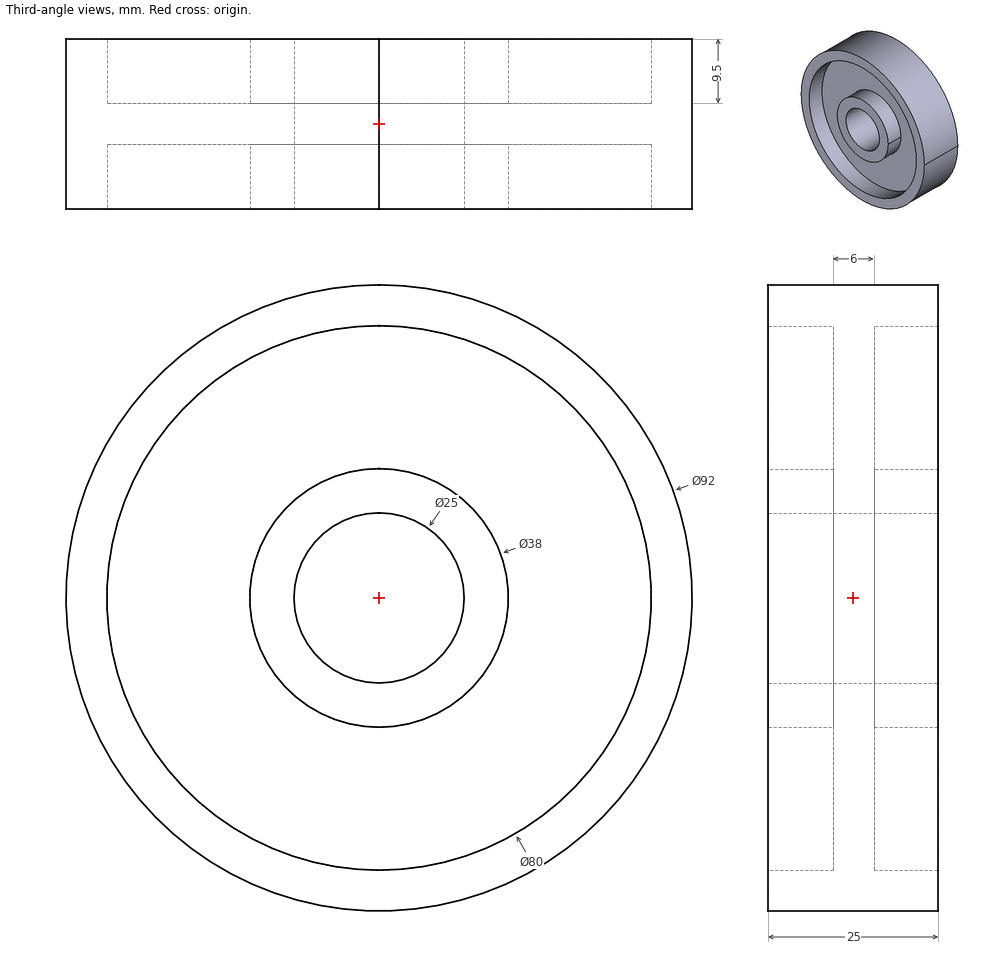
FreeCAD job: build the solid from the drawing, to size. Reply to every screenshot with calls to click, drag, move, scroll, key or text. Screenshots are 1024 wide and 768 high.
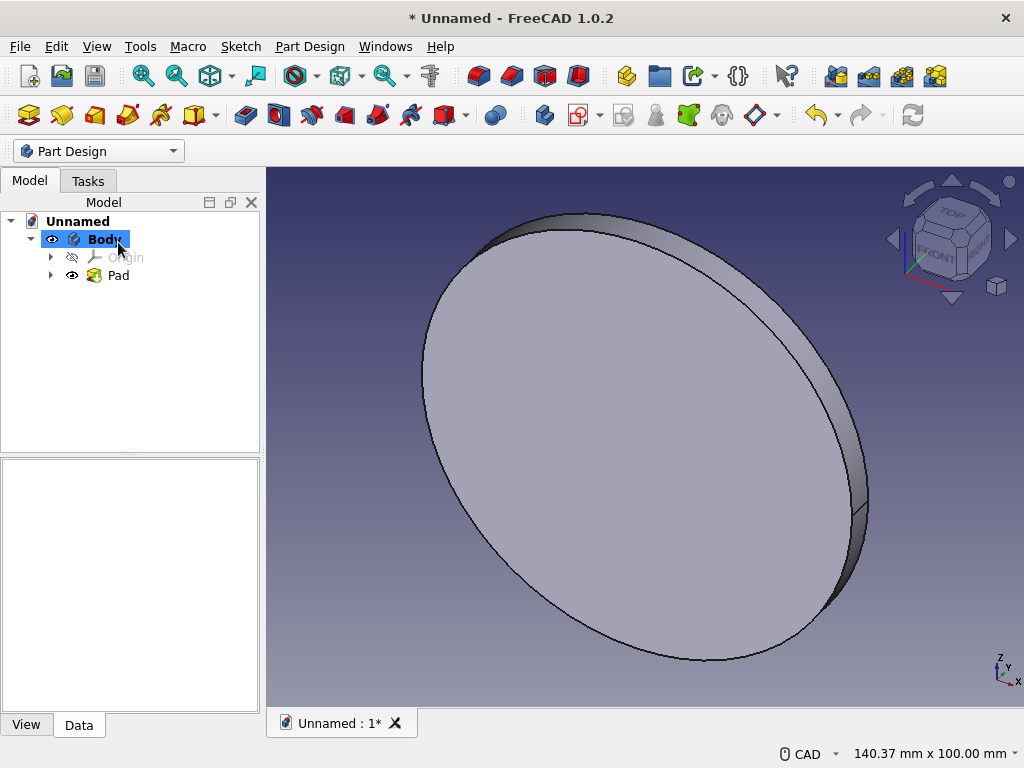
key(v)
key(f)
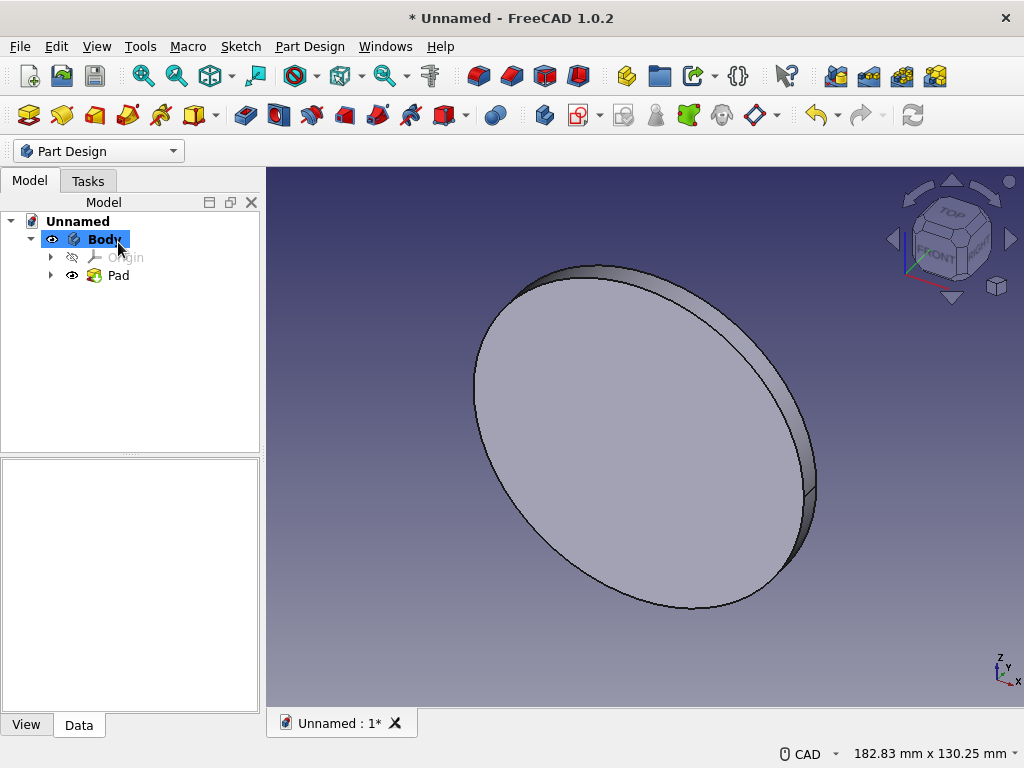
click(51, 257)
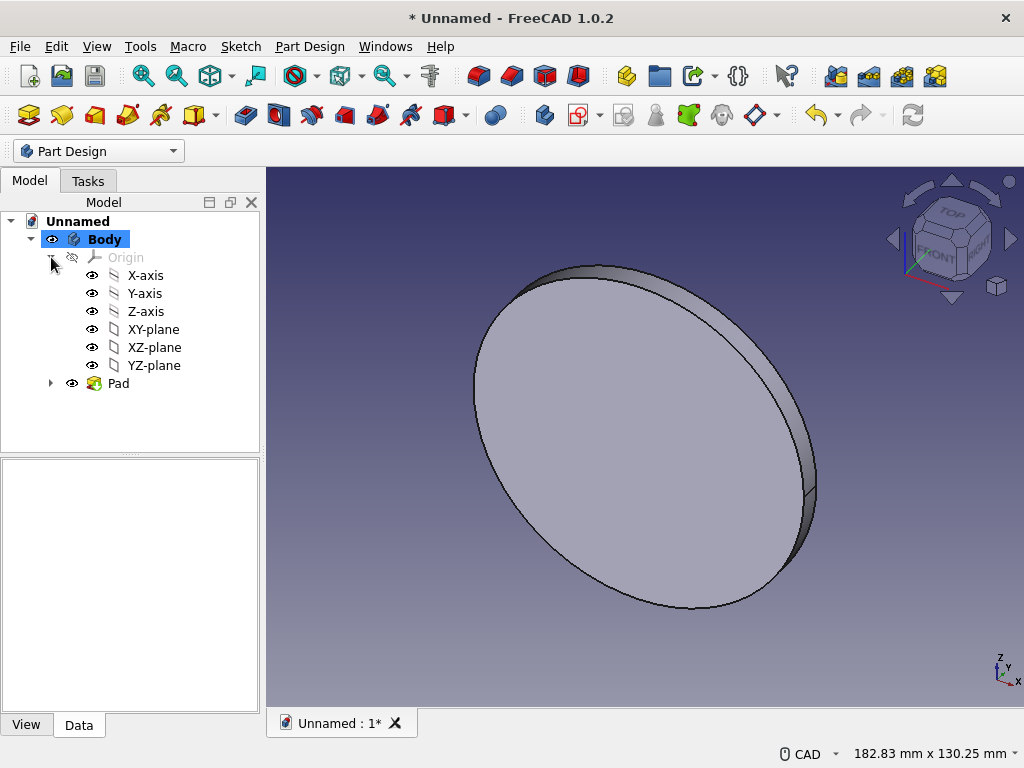
click(137, 347)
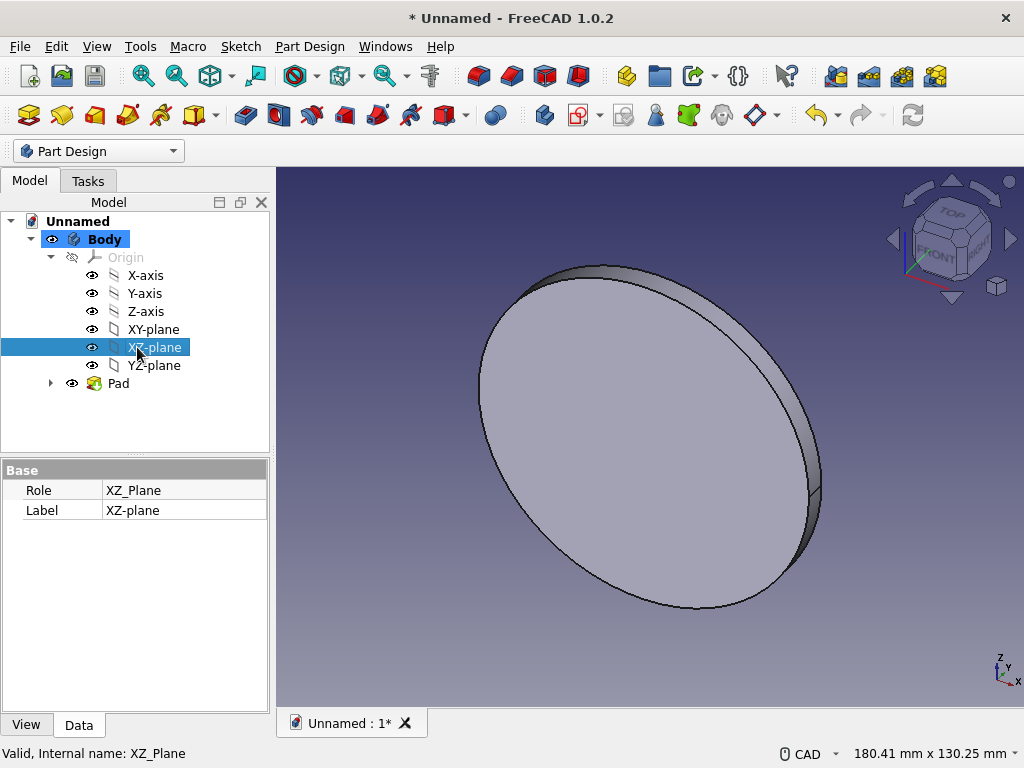
click(754, 116)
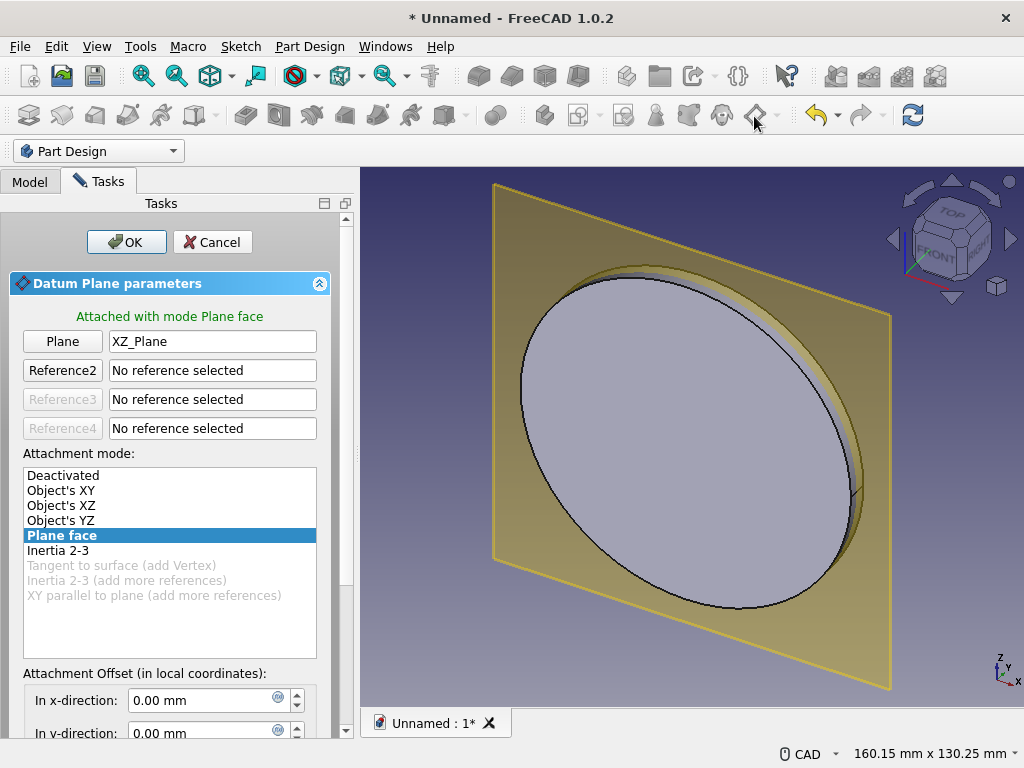
scroll(346, 476, down, 2)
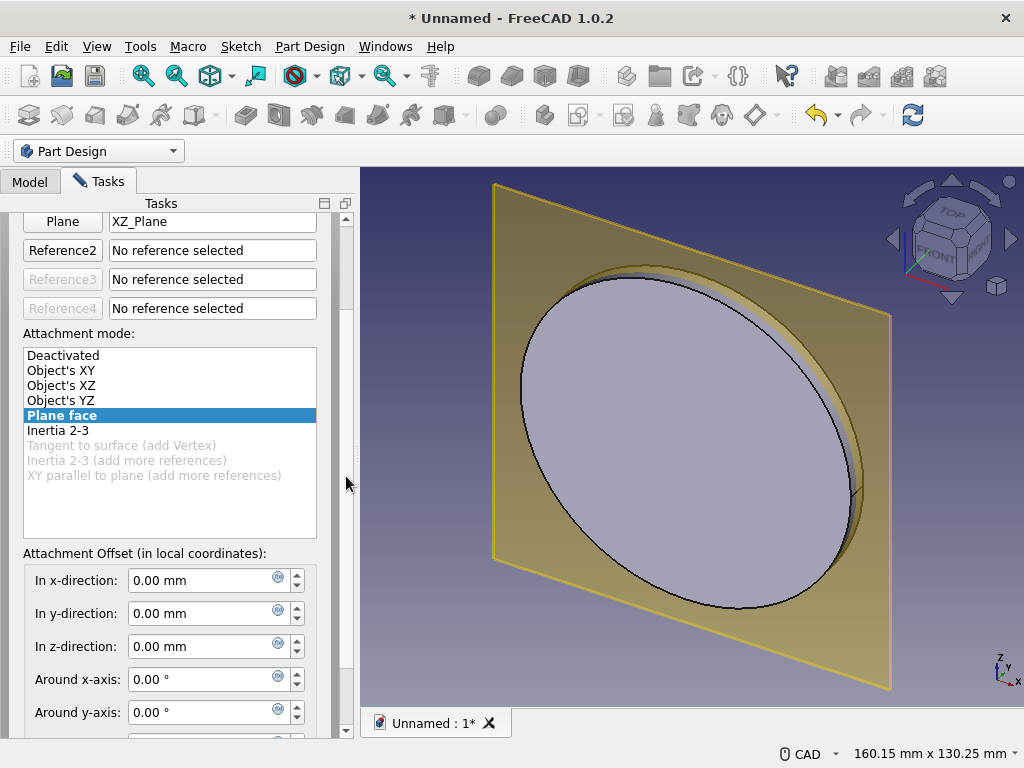
triple_click(210, 646)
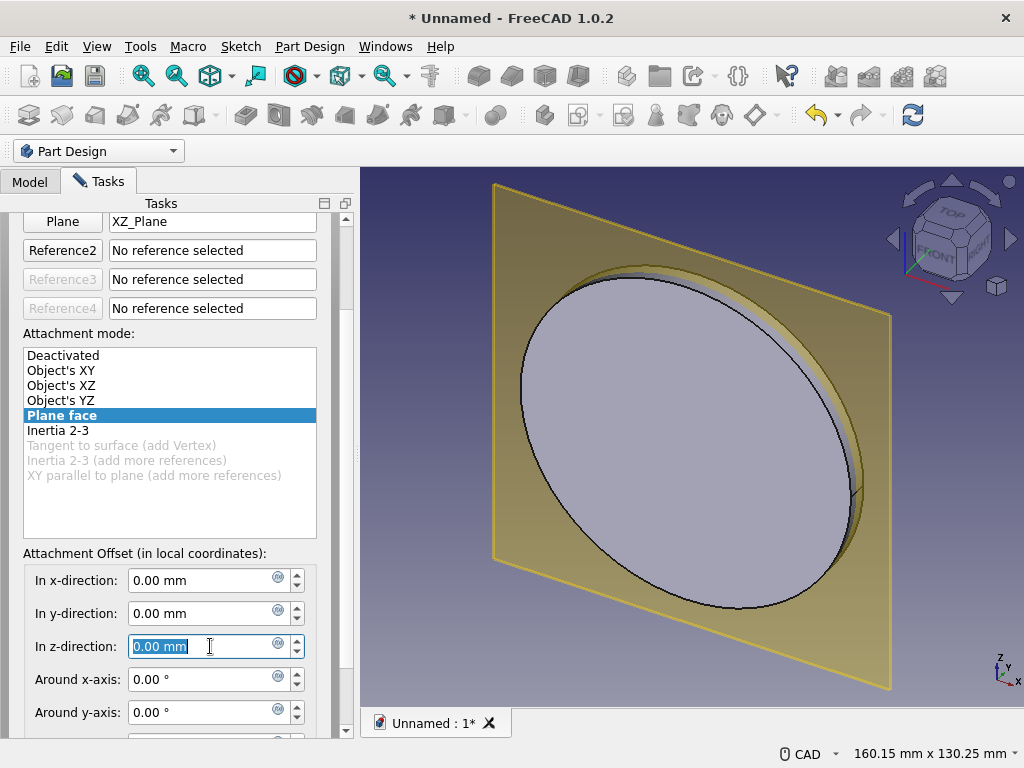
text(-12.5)
key(Tab)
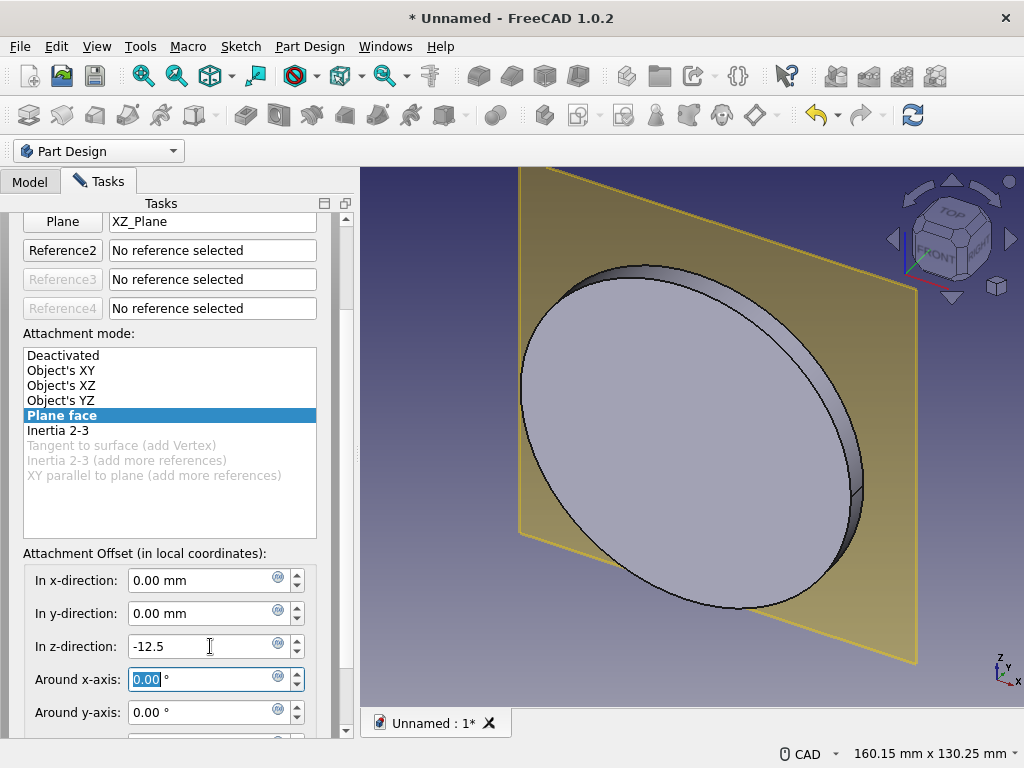
scroll(346, 476, up, 3)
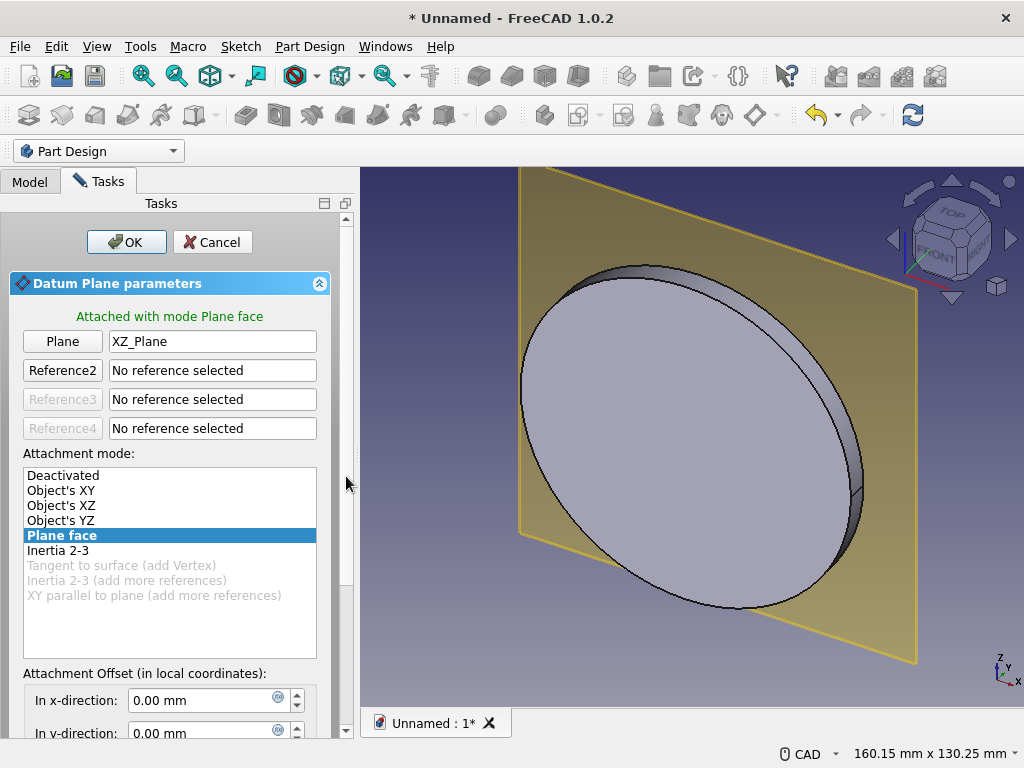
click(127, 242)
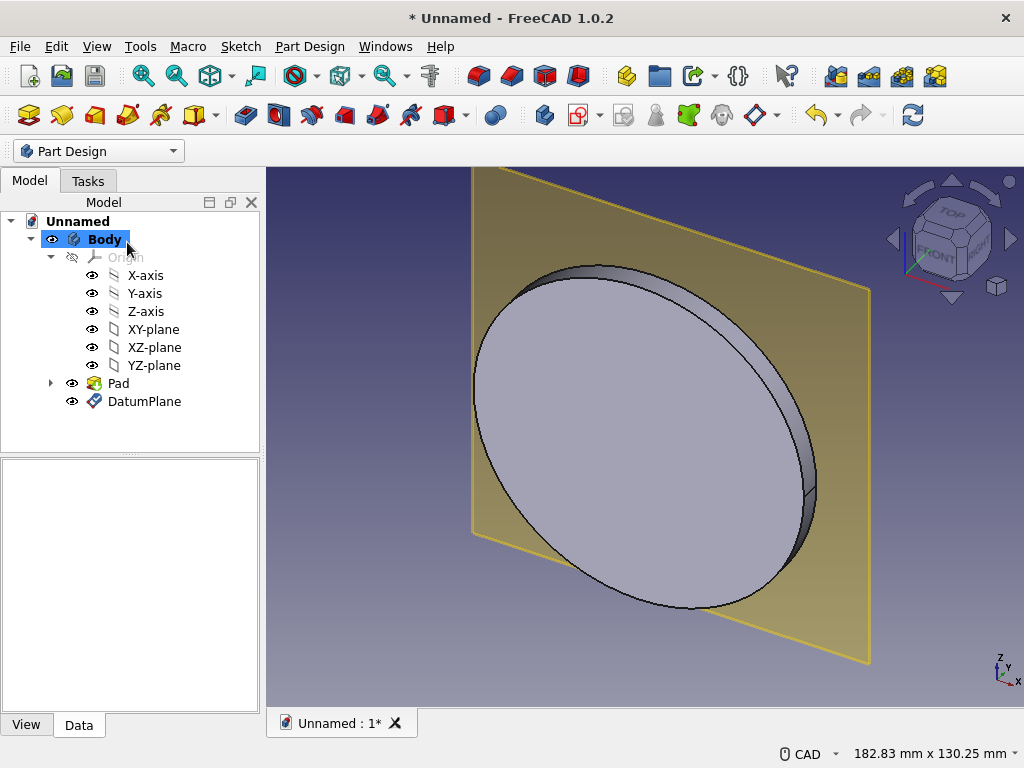
click(117, 401)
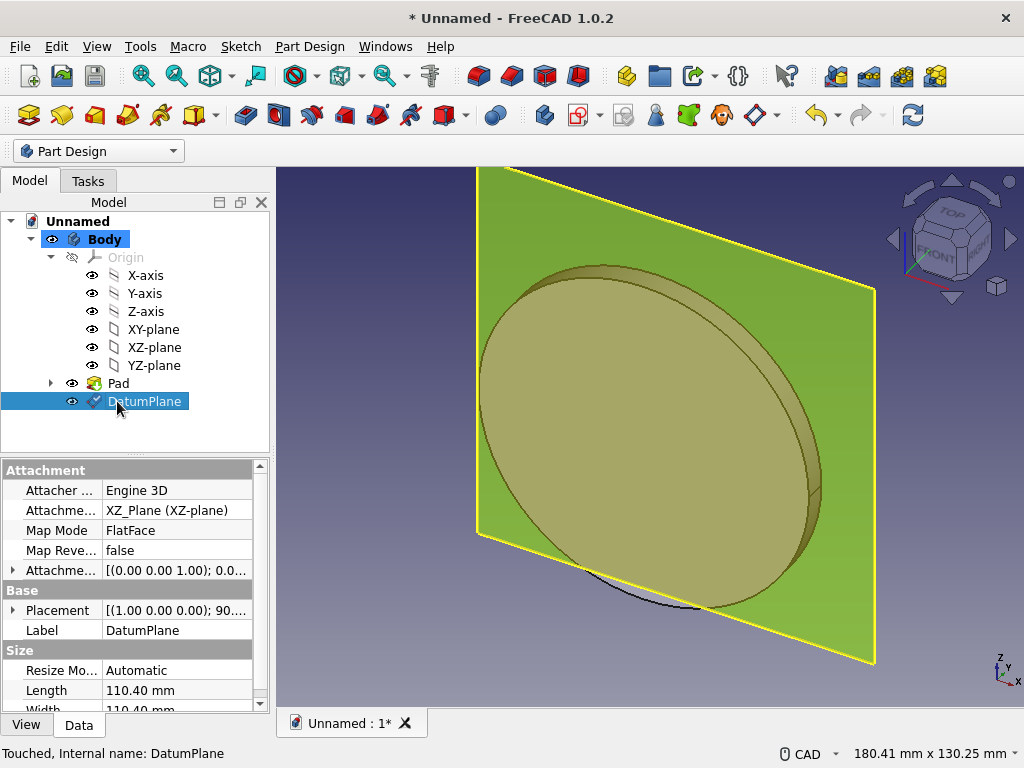
click(578, 116)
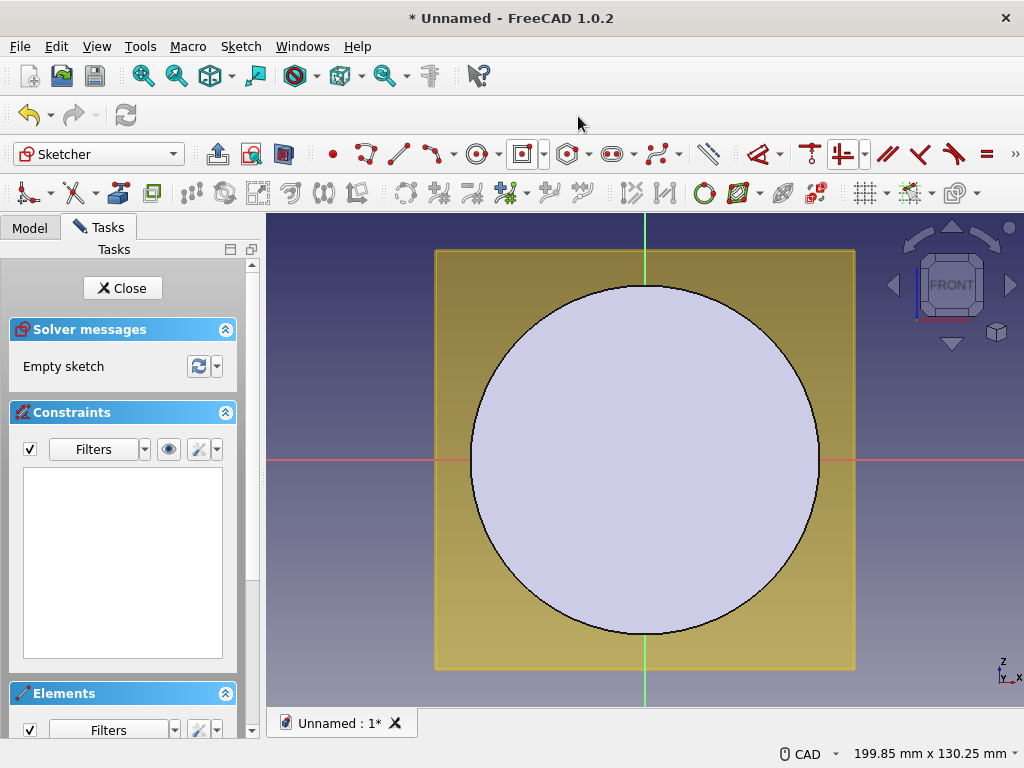
key(q)
key(s)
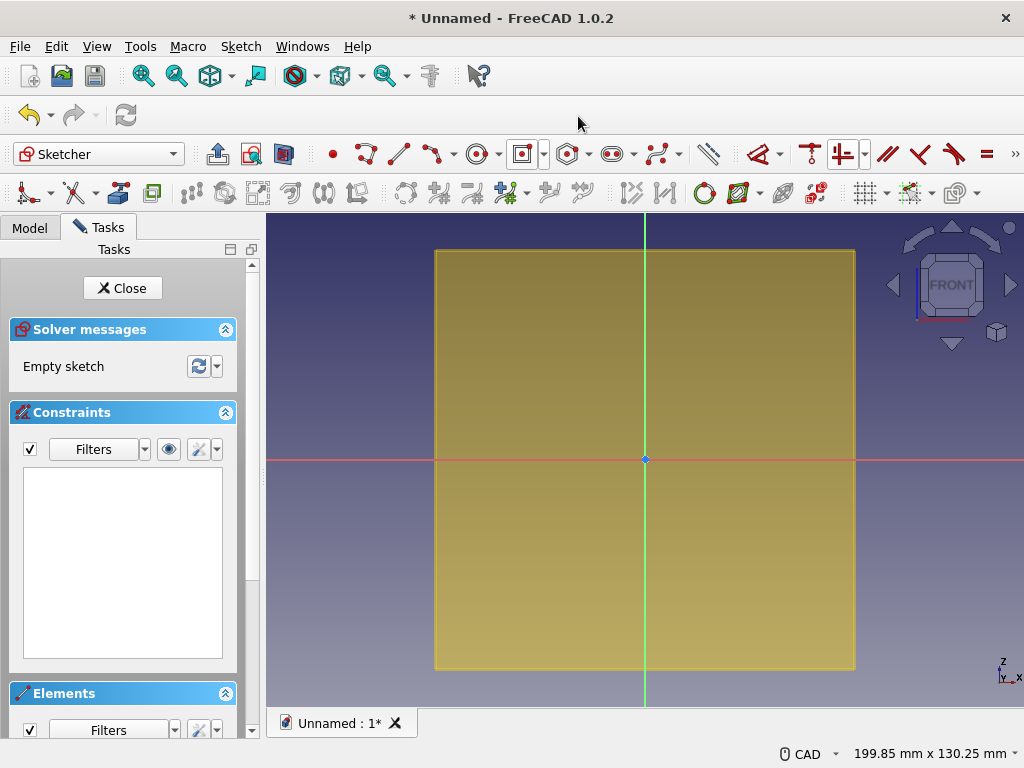
key(g)
key(c)